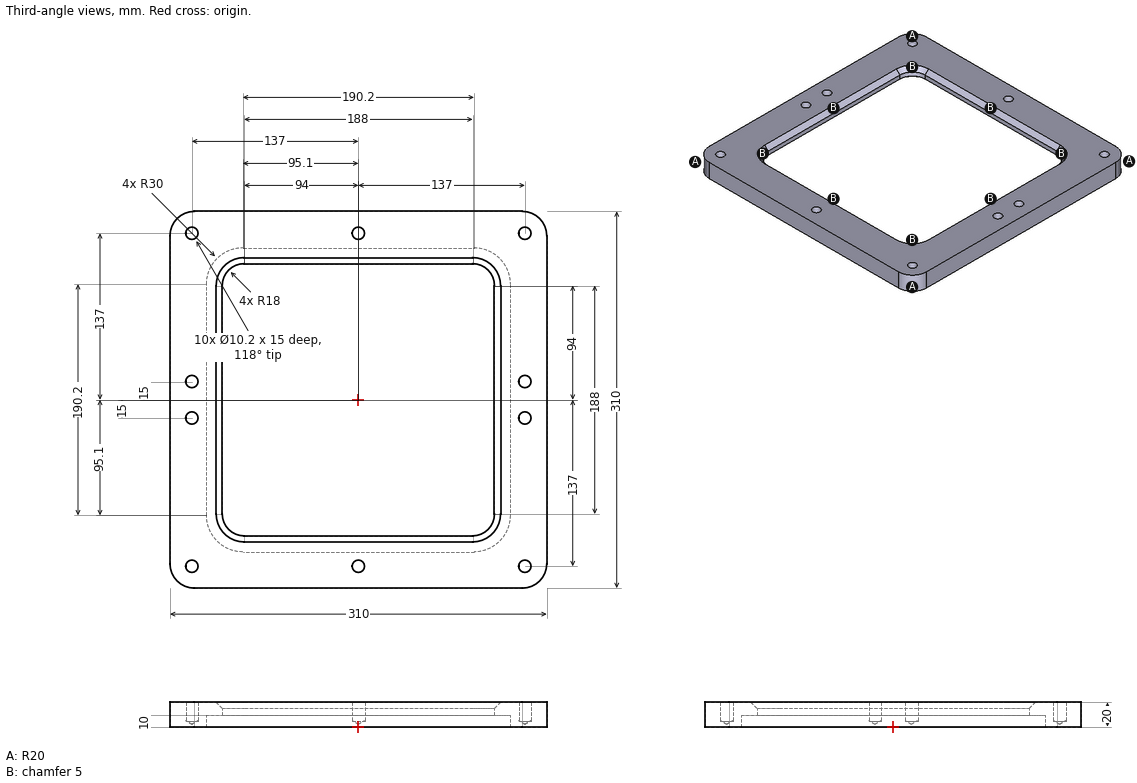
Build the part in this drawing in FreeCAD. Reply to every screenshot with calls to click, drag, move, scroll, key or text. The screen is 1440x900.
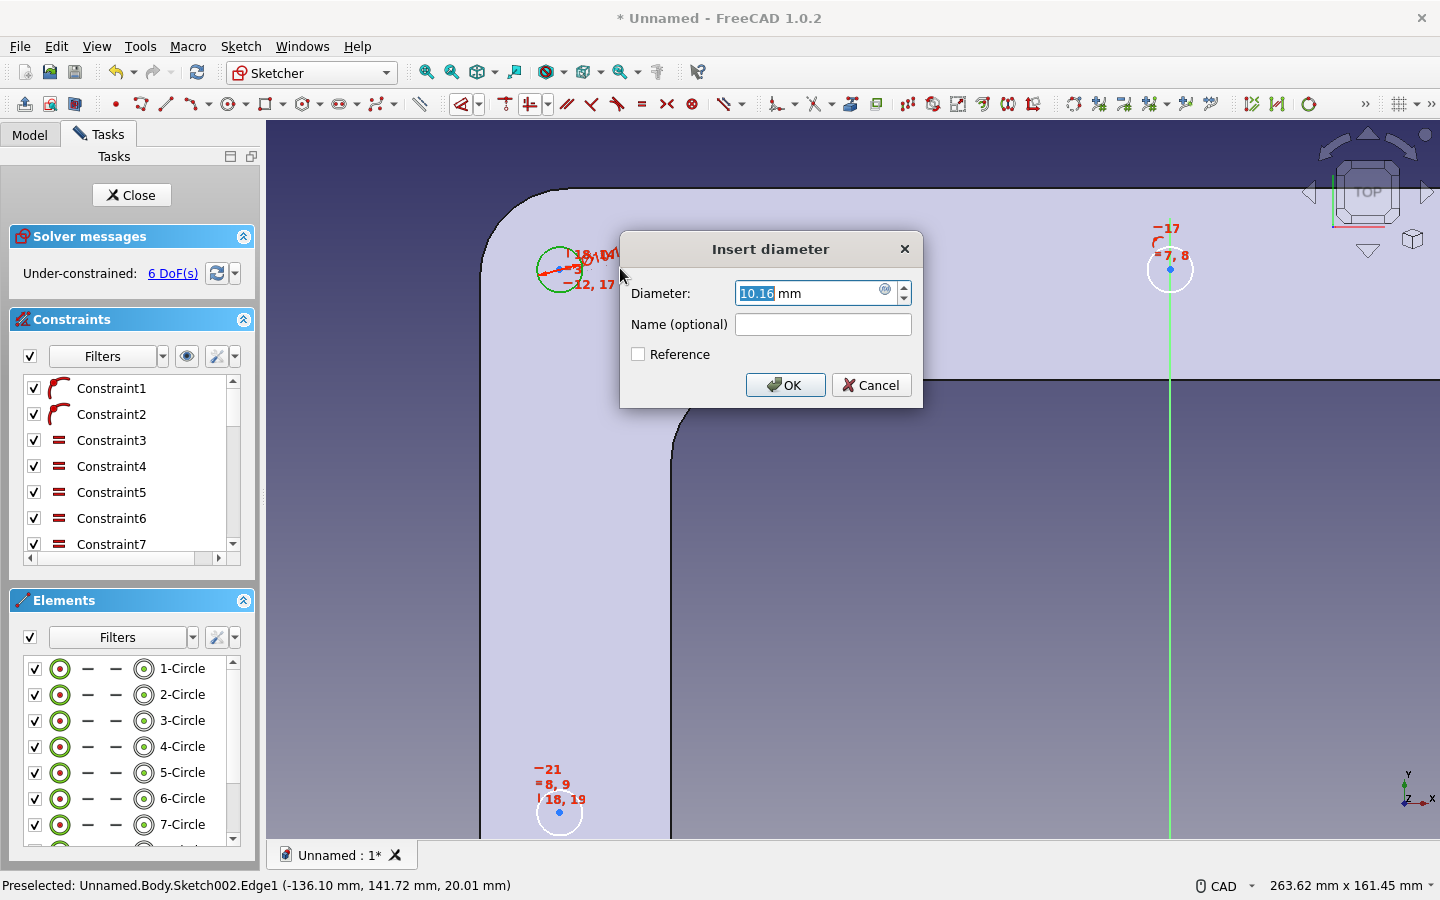
text(10.2)
key(Return)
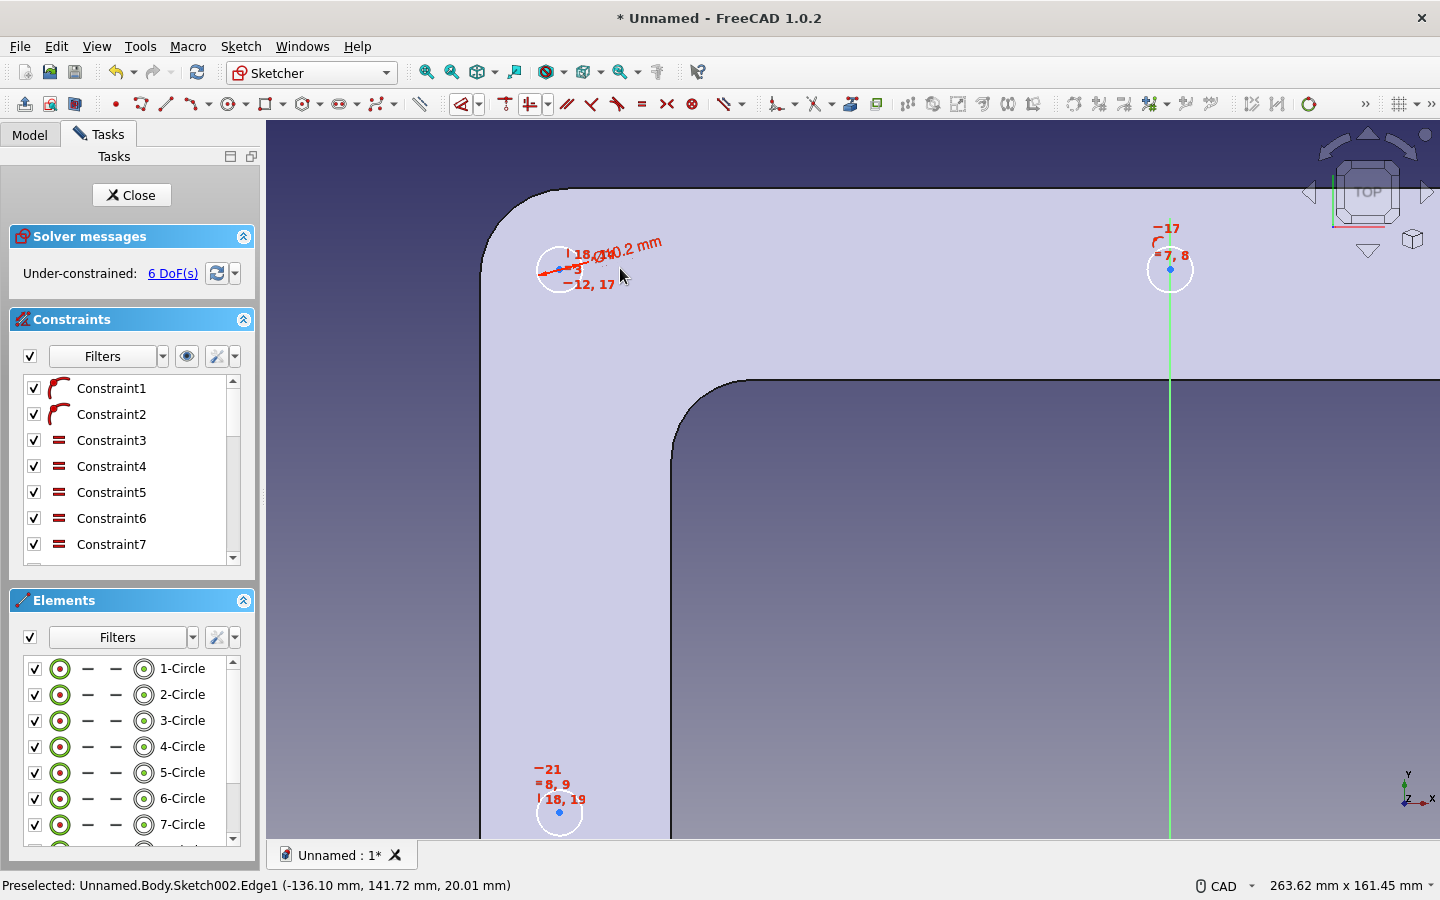
scroll(560, 247, down, 5)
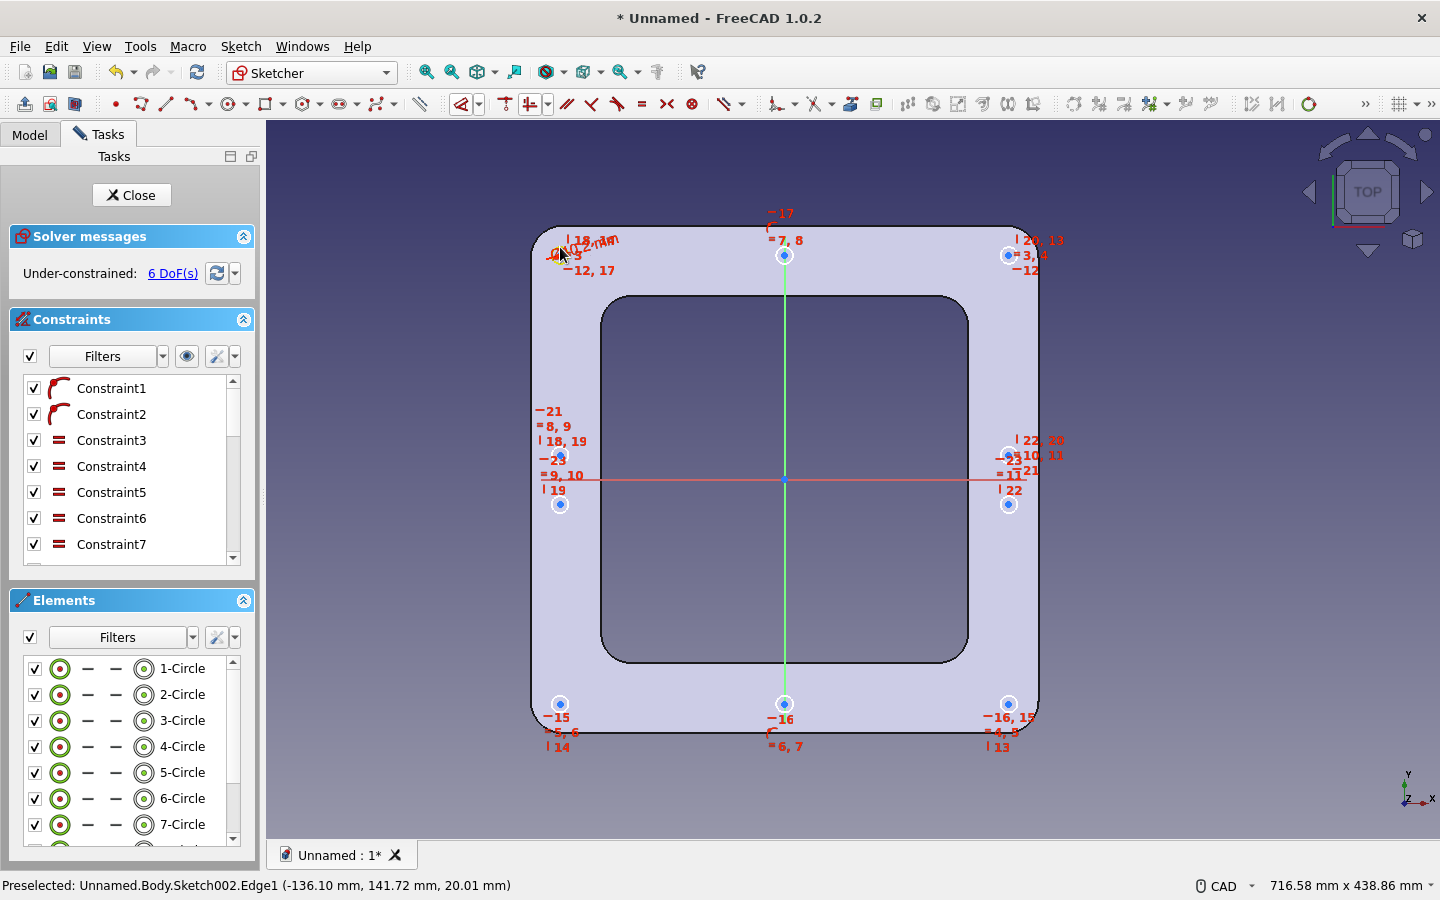
scroll(560, 455, up, 3)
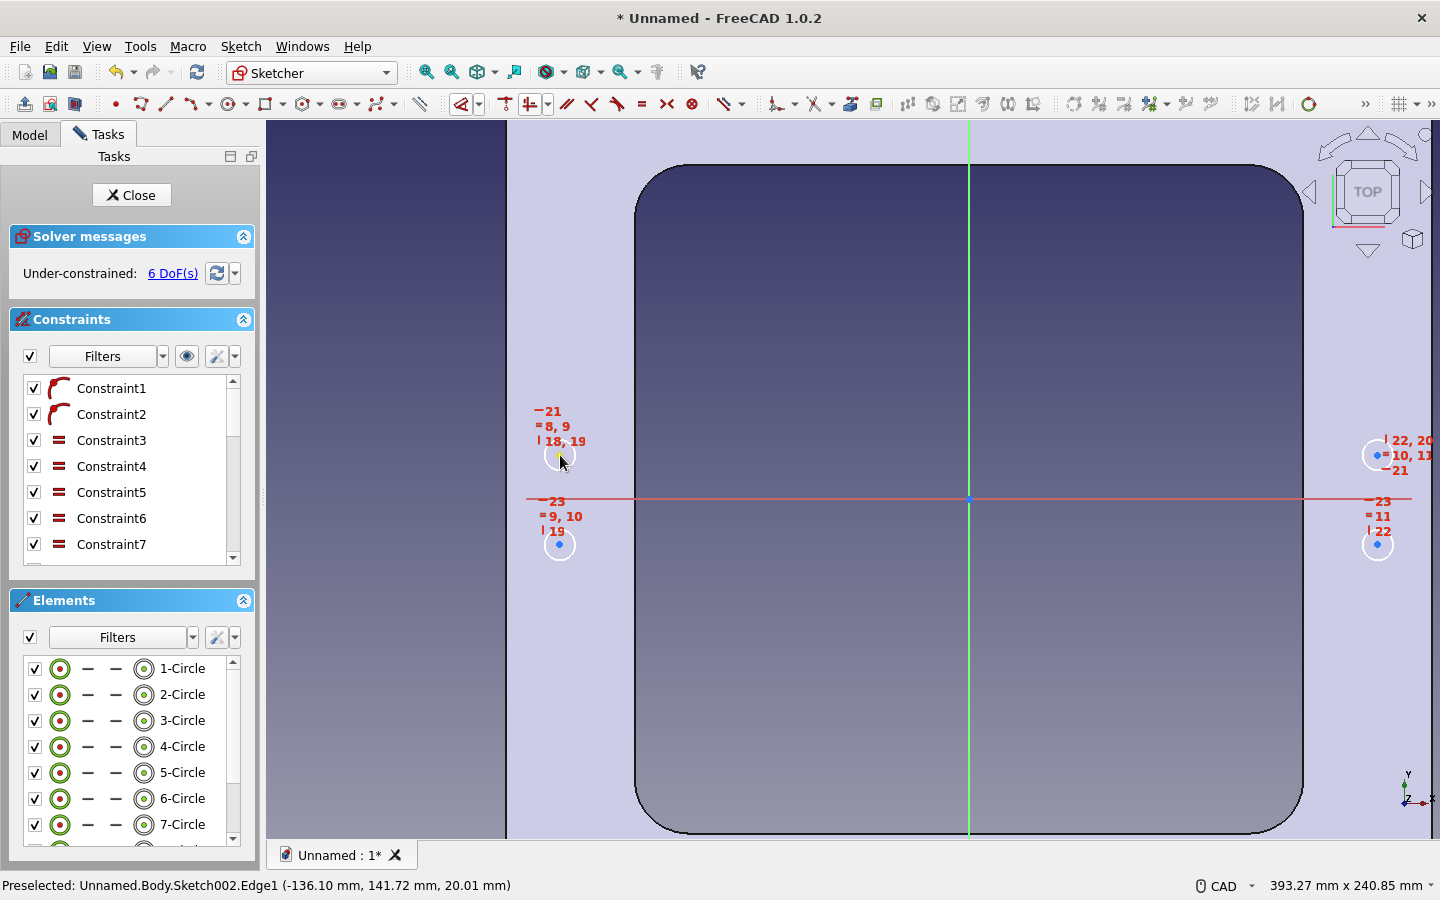
click(560, 455)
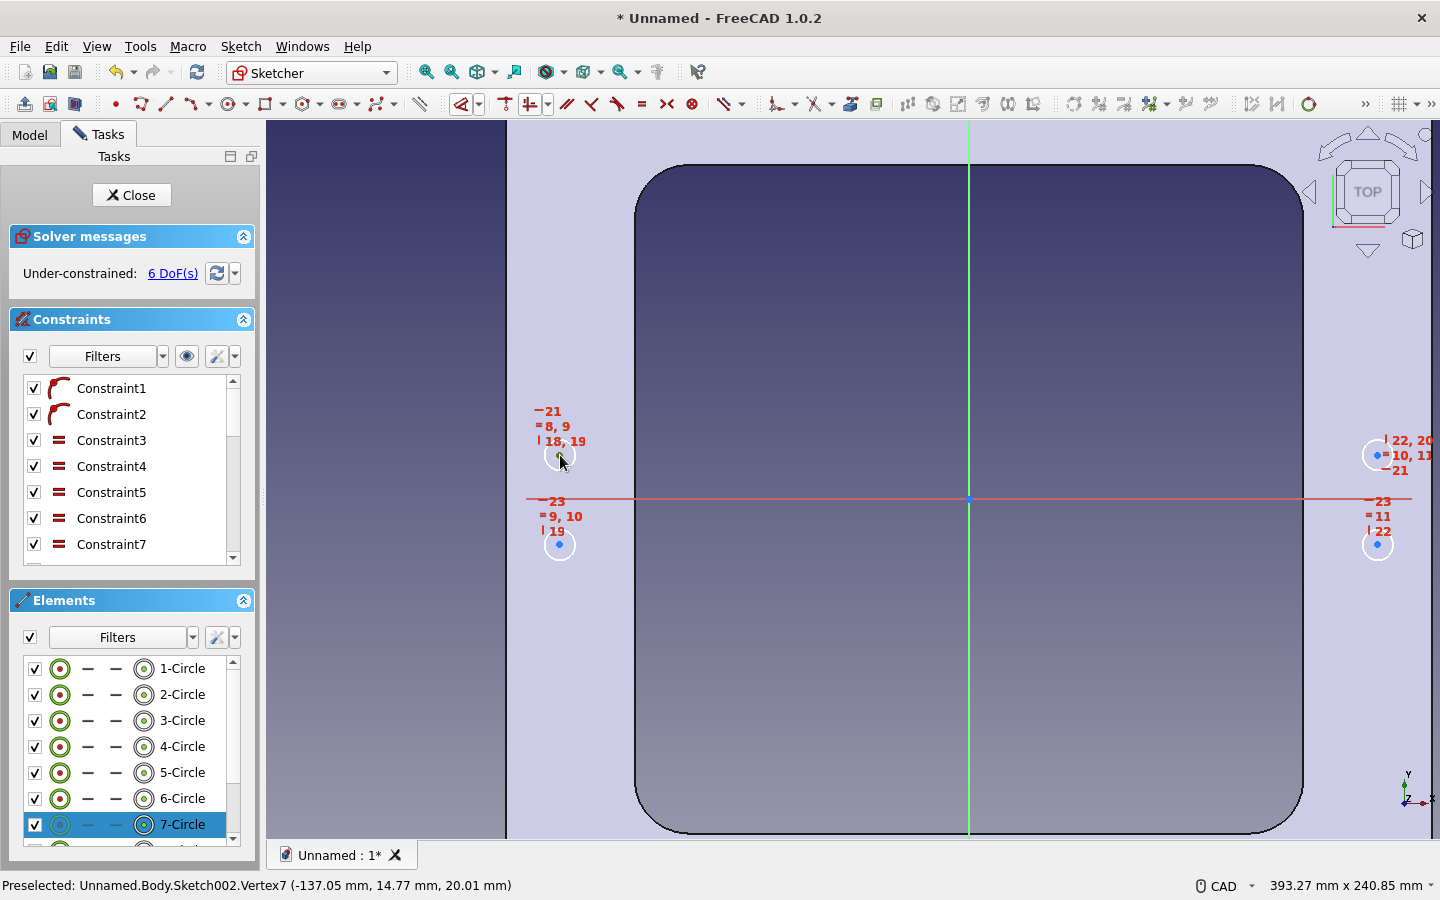
click(478, 104)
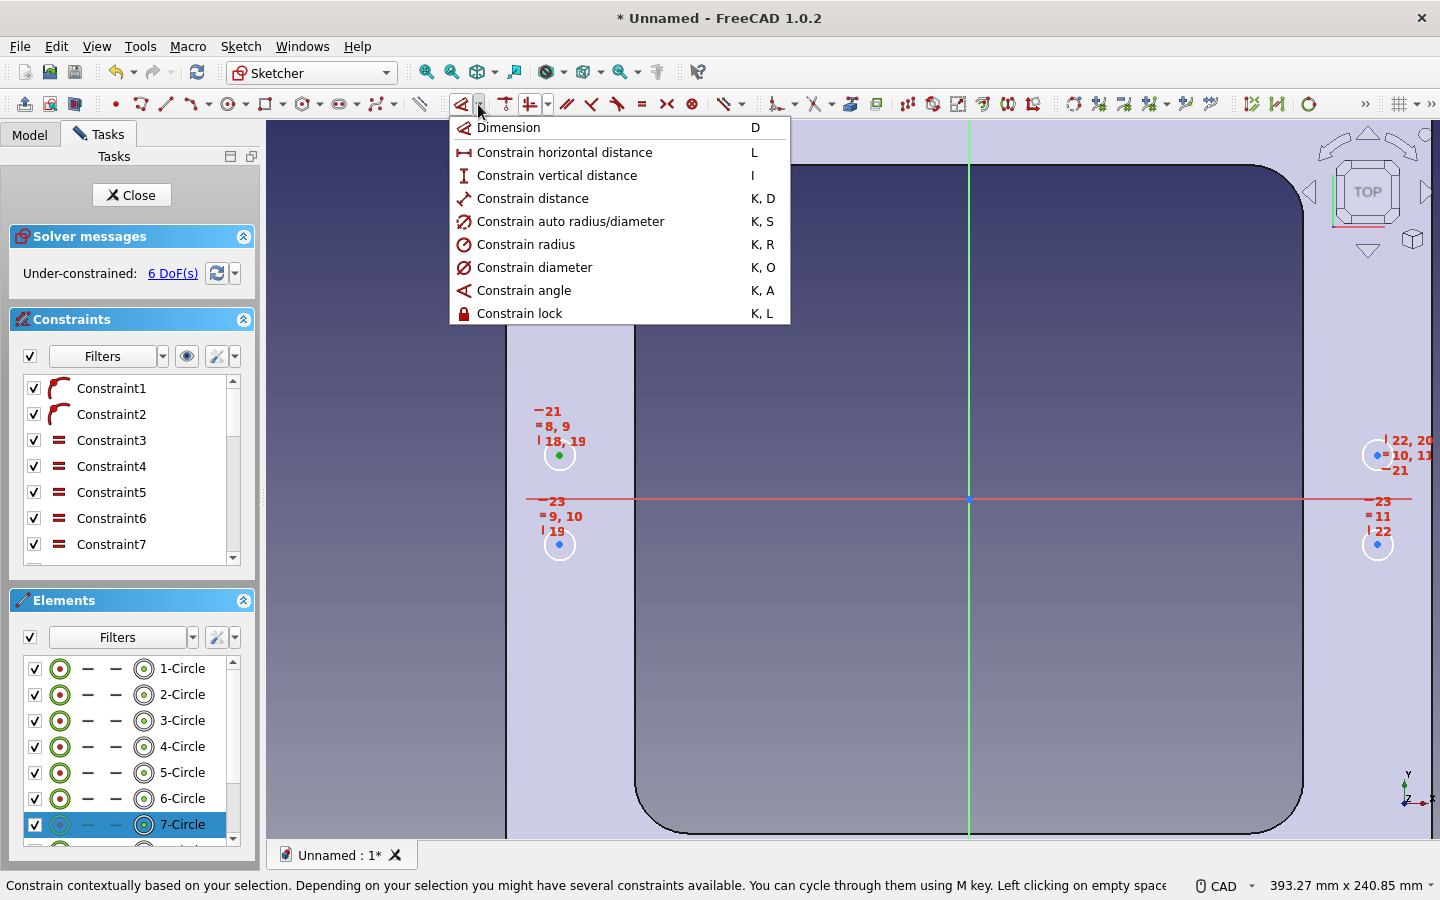
click(620, 176)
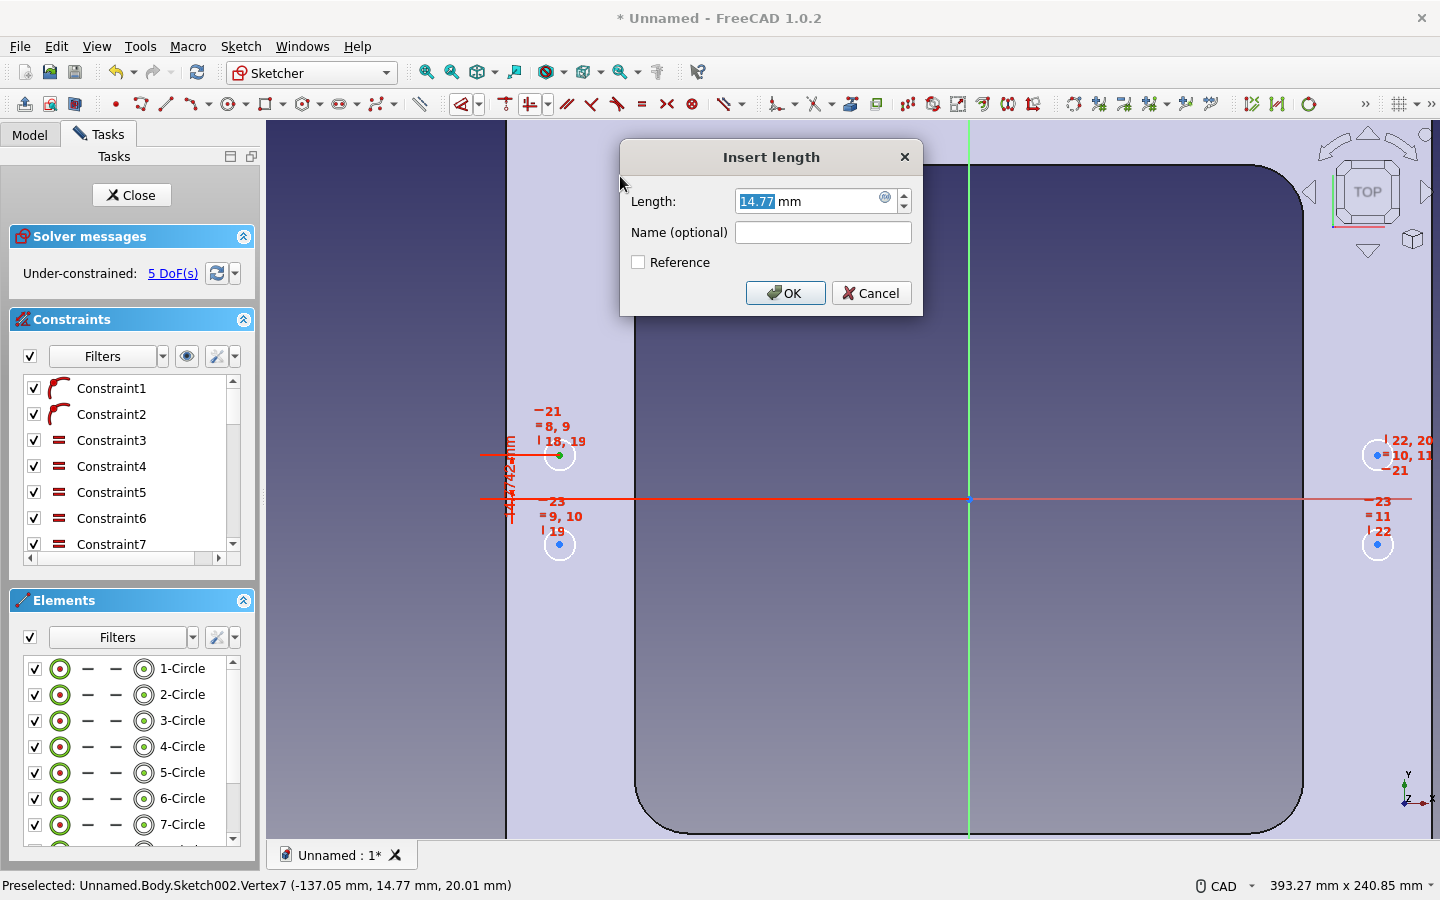
text(15)
key(Return)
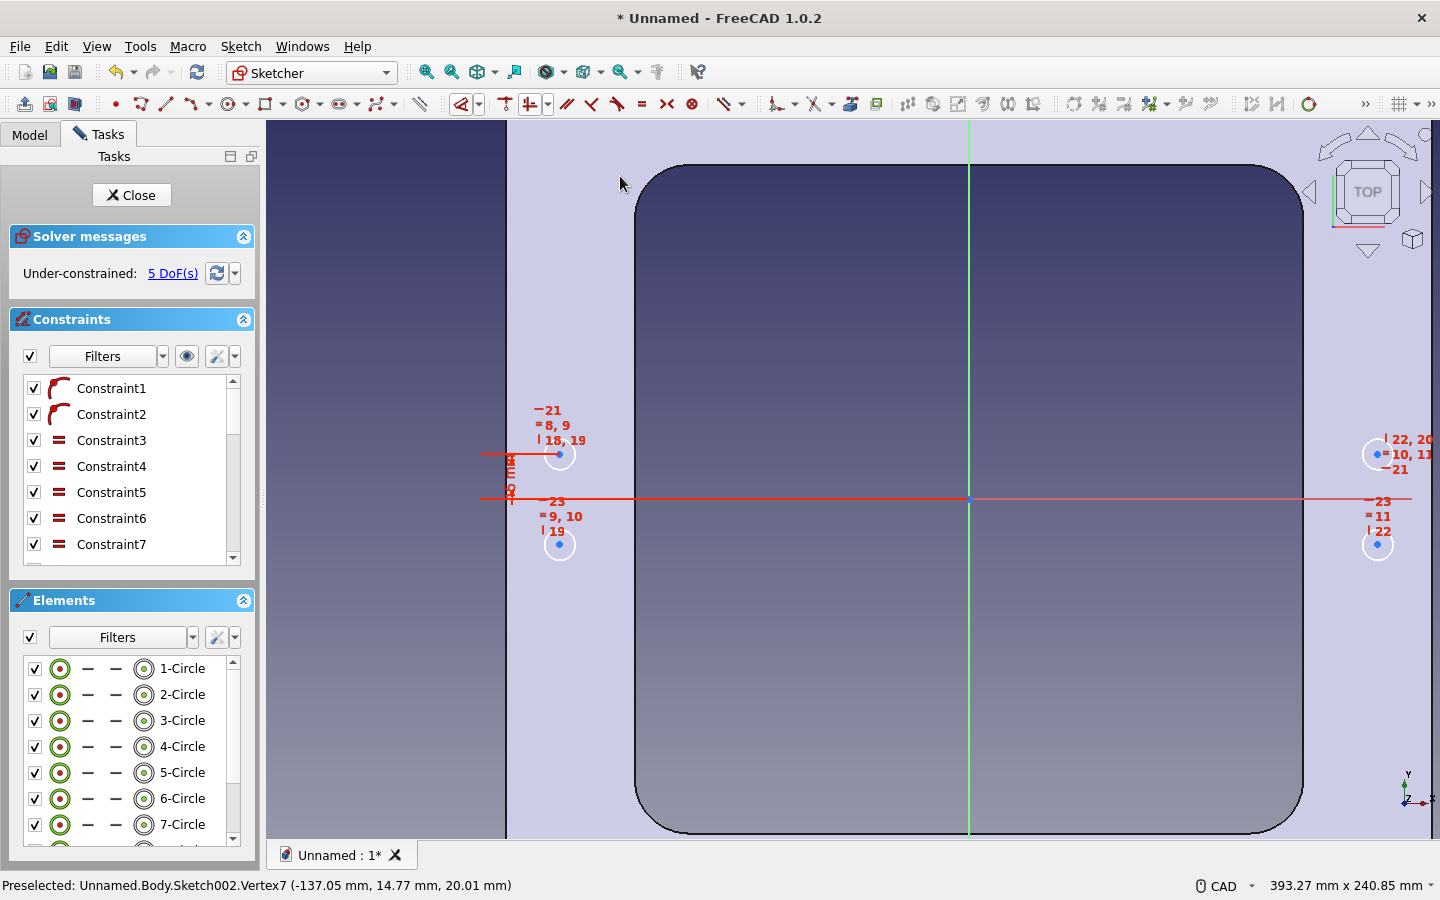
click(560, 545)